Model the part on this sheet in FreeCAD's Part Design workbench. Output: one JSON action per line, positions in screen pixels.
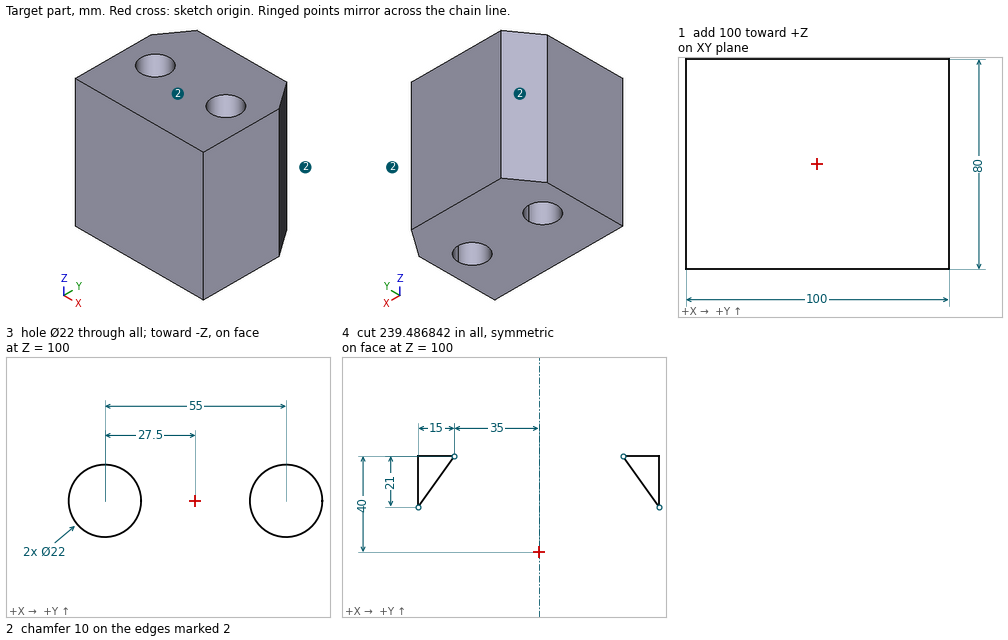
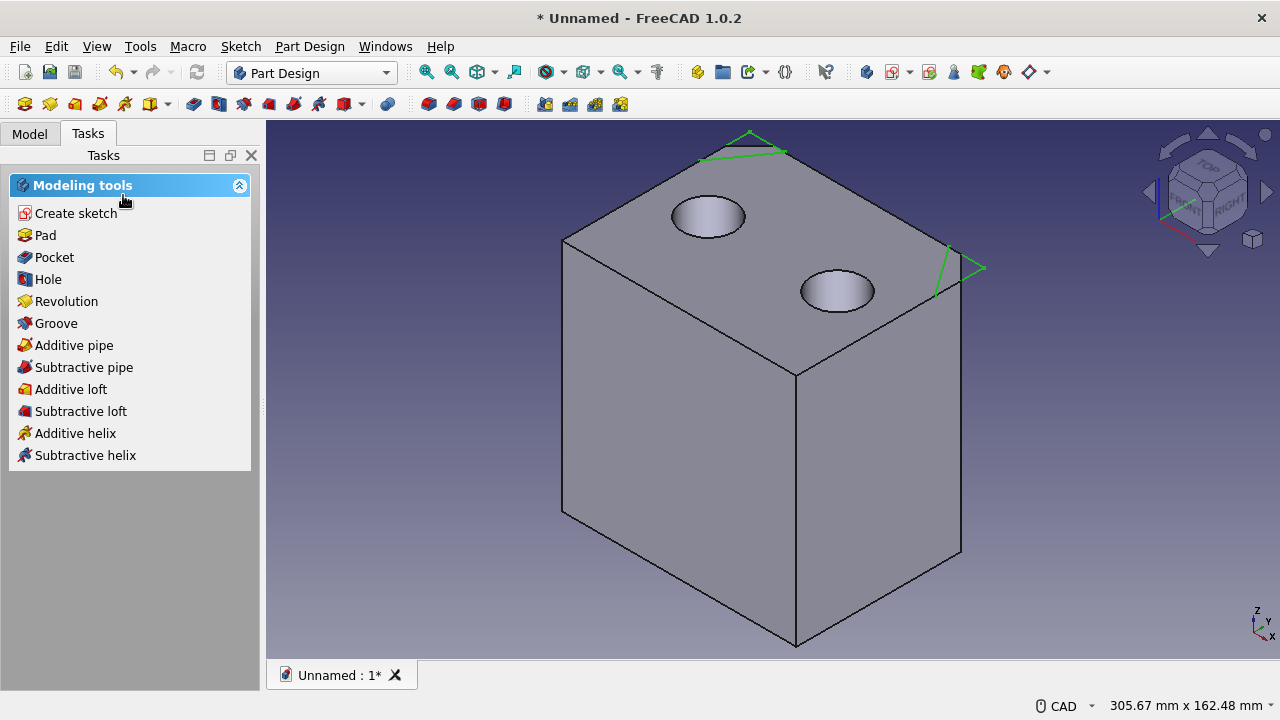
{"action": "left_click", "coordinate": [194, 104]}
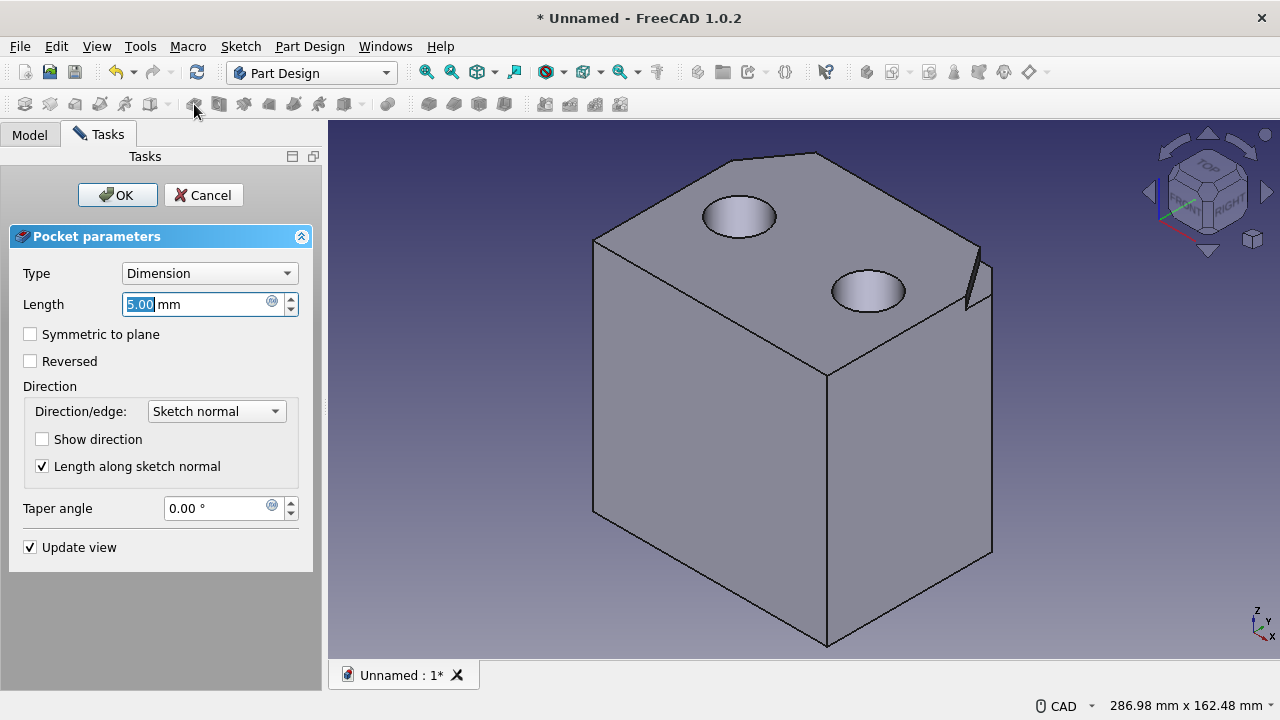
{"action": "type", "text": "239.486842"}
{"action": "key", "text": "Tab"}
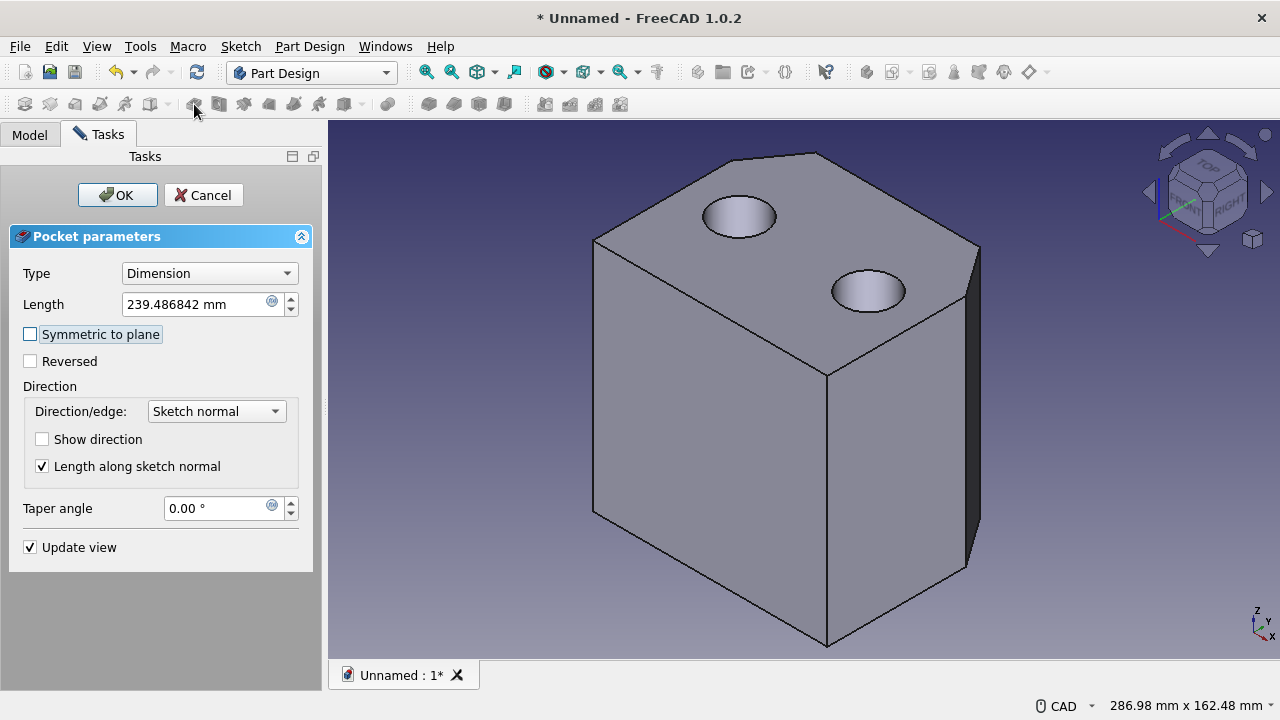
{"action": "left_click", "coordinate": [31, 334]}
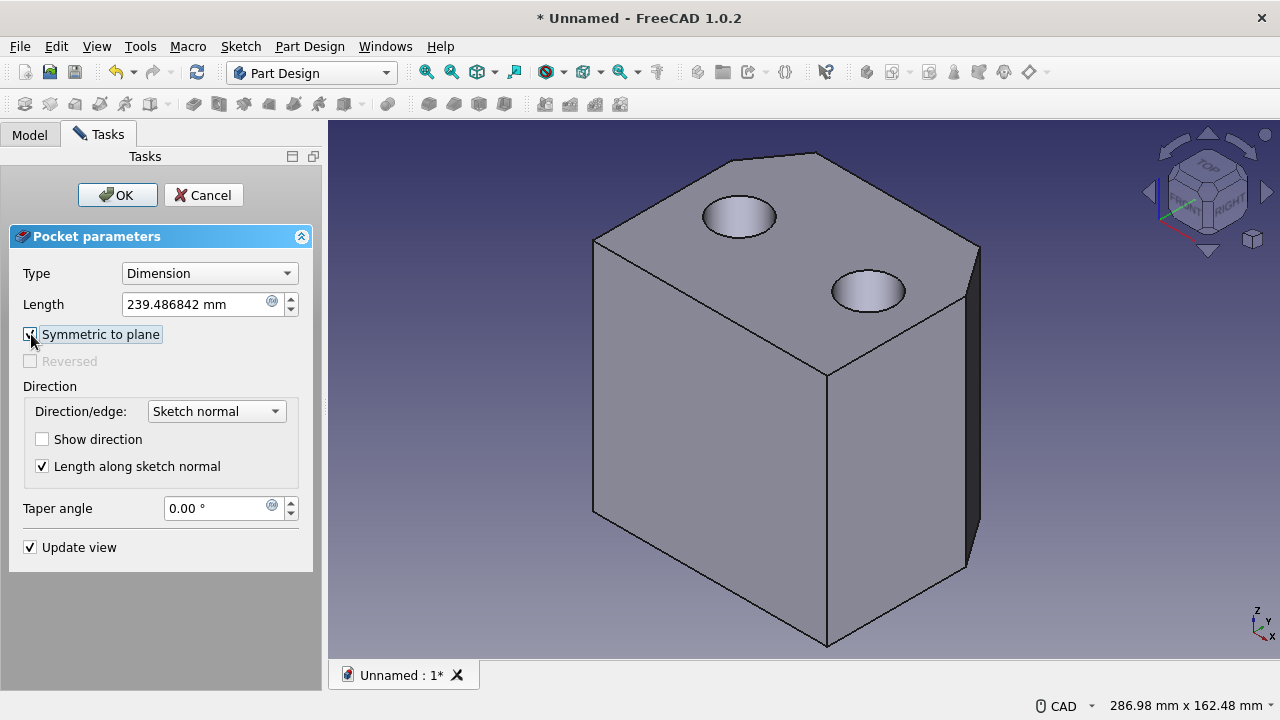
{"action": "left_click", "coordinate": [118, 195]}